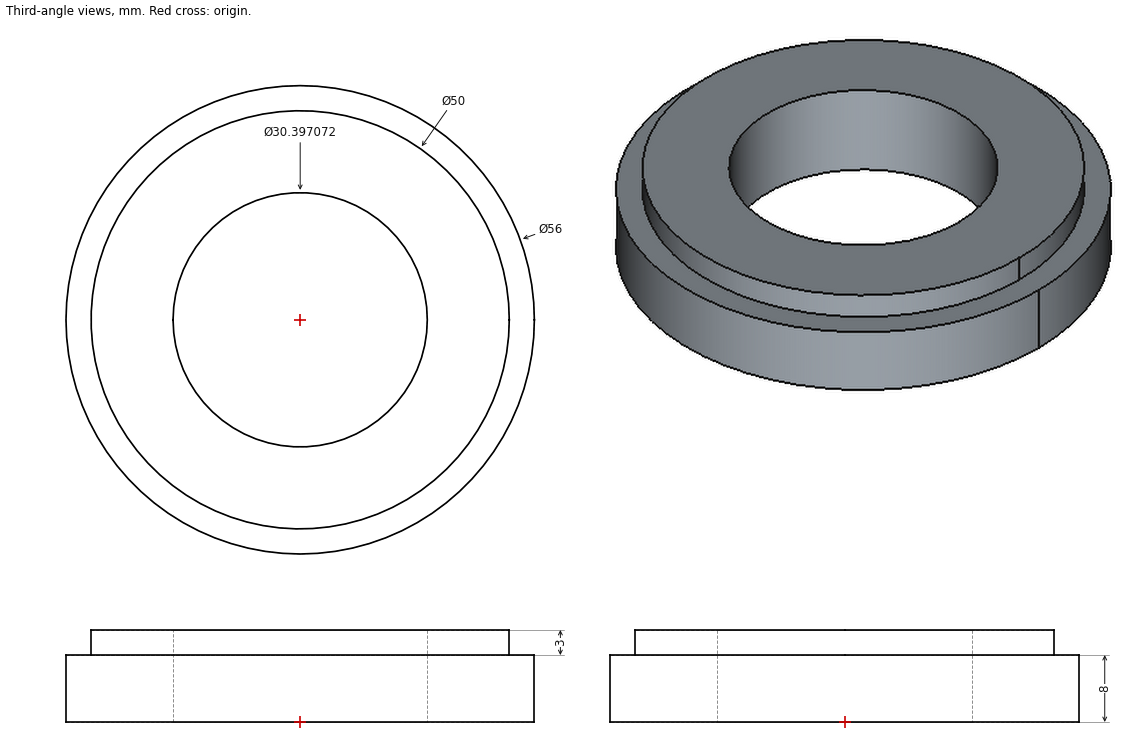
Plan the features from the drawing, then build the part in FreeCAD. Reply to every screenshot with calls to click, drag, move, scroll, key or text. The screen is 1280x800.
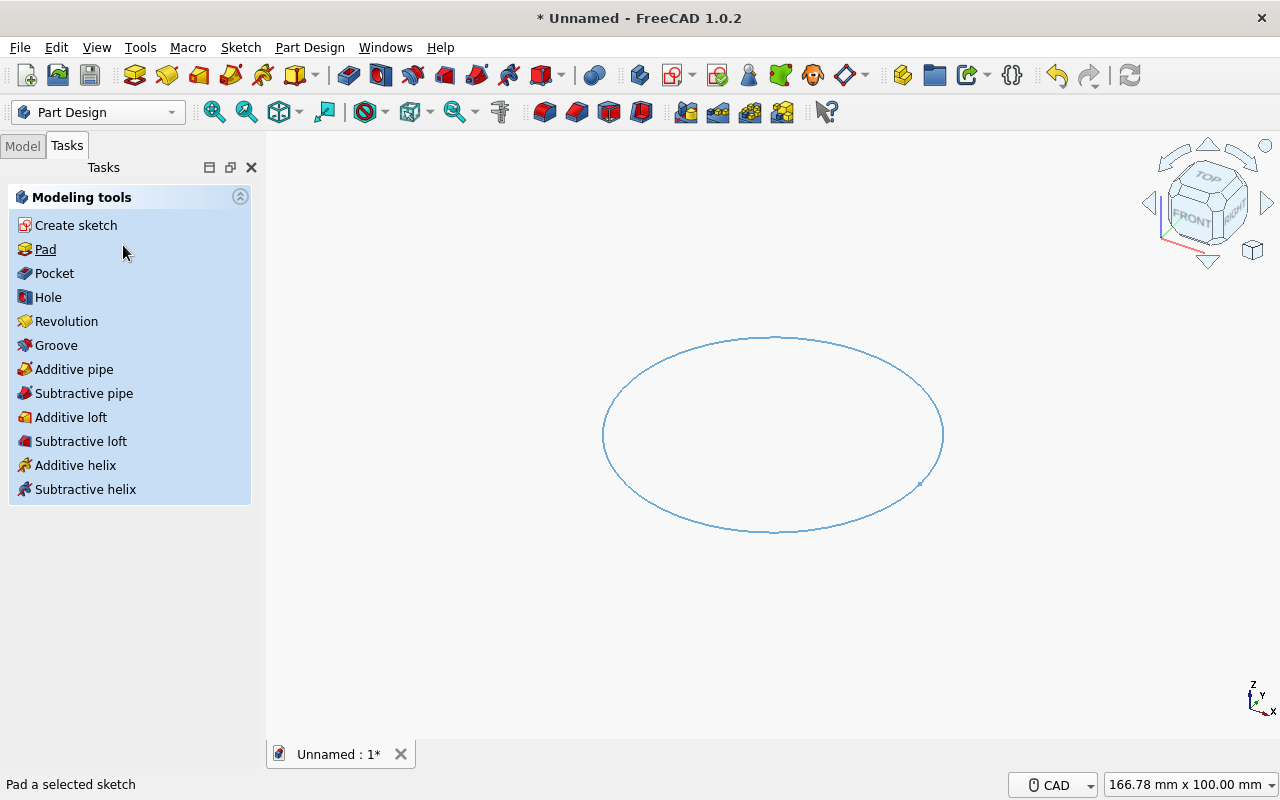
click(136, 76)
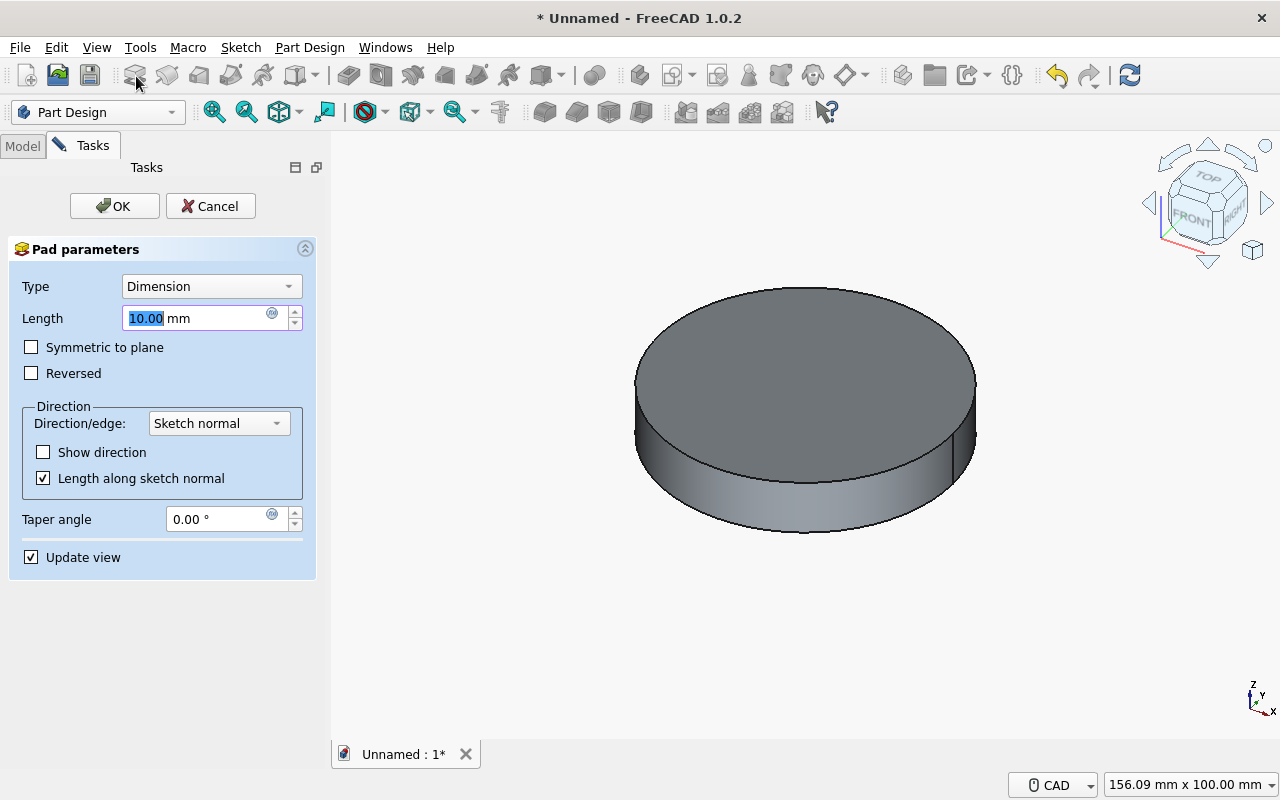
text(8)
key(Tab)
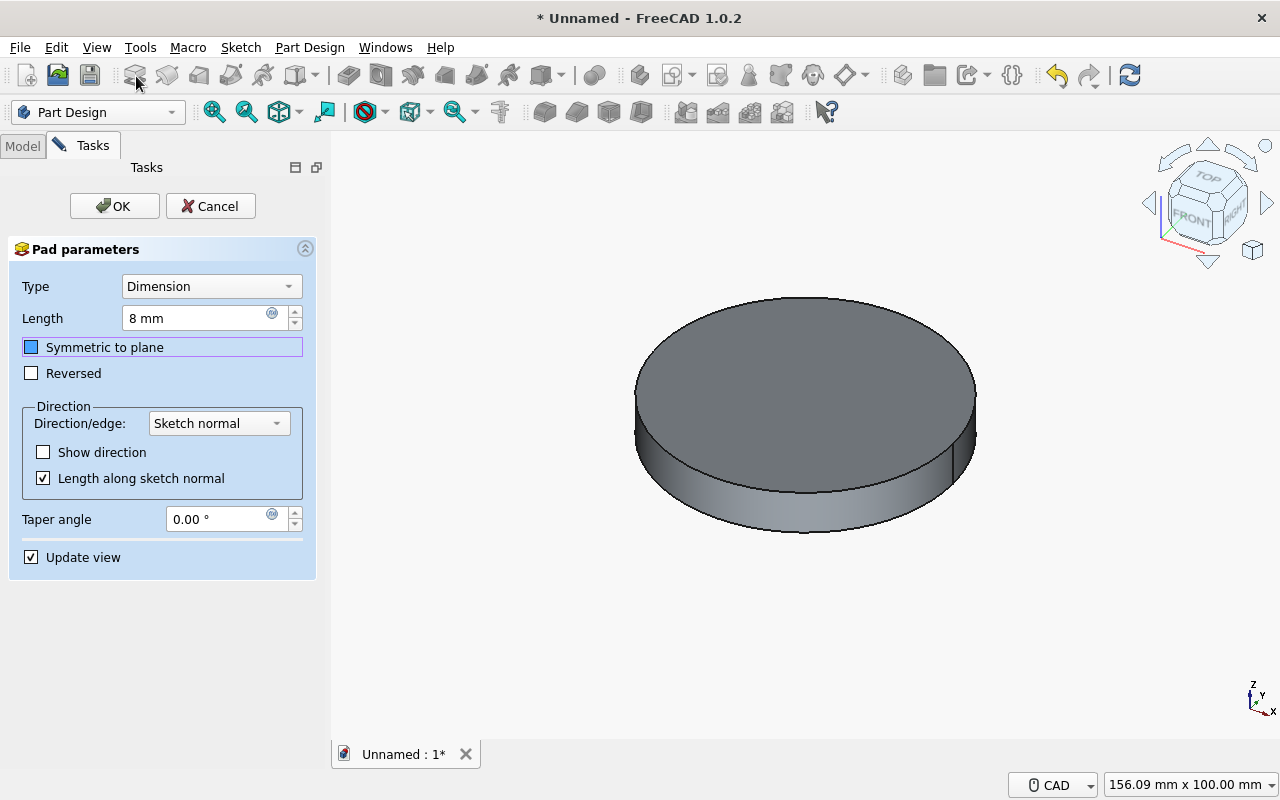
click(115, 206)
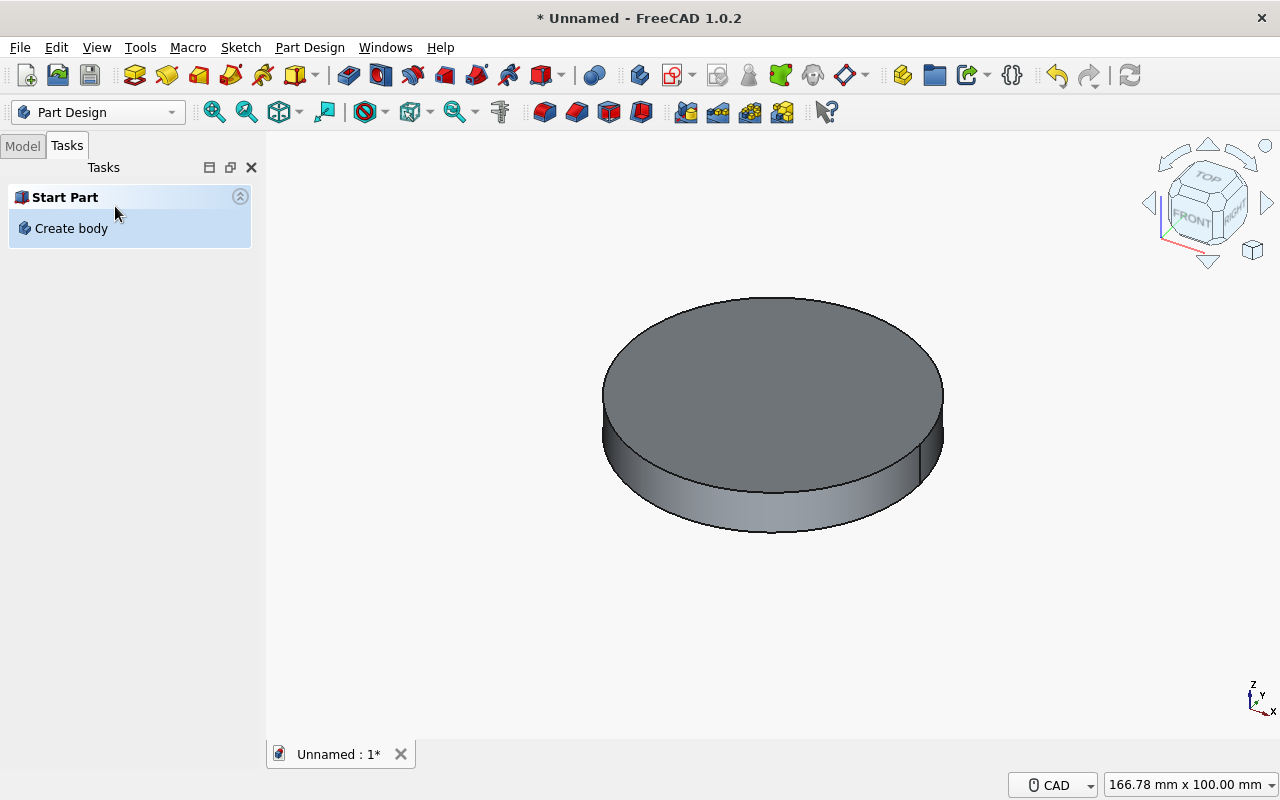
click(773, 394)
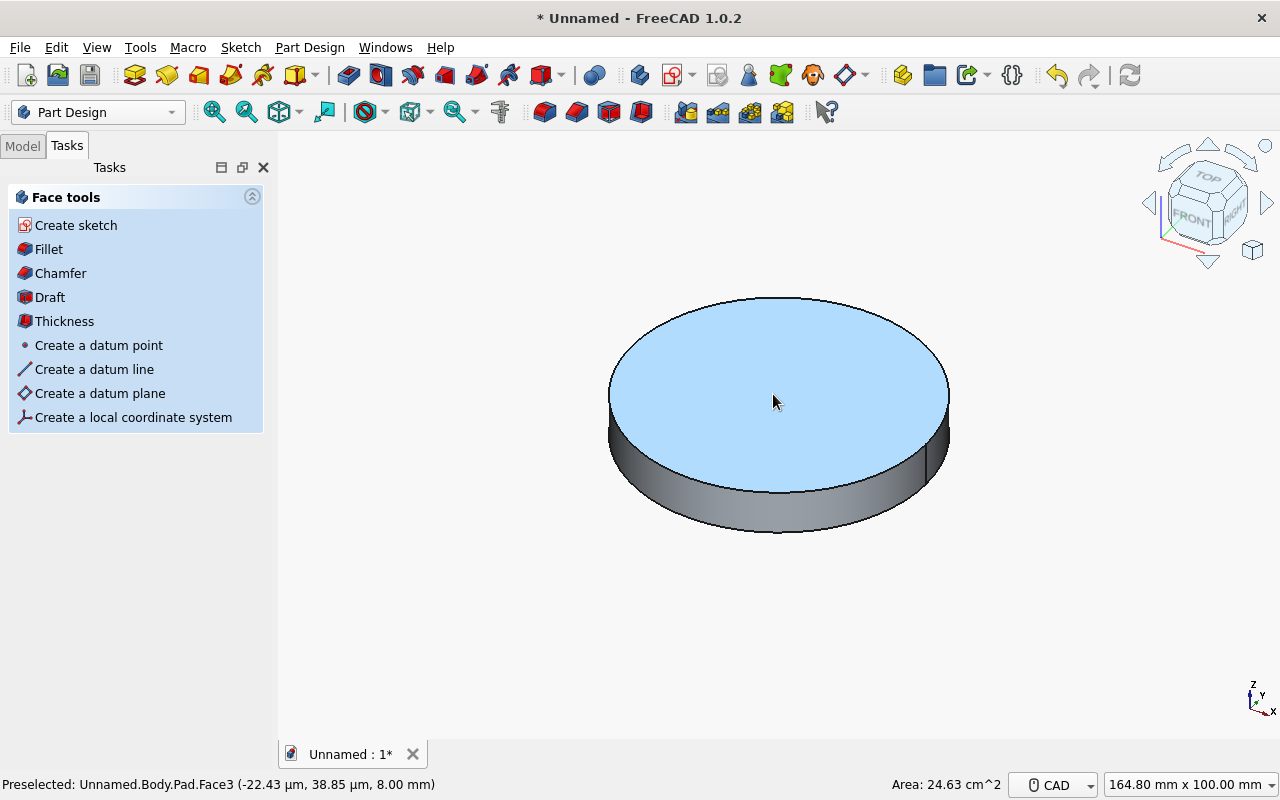
click(672, 76)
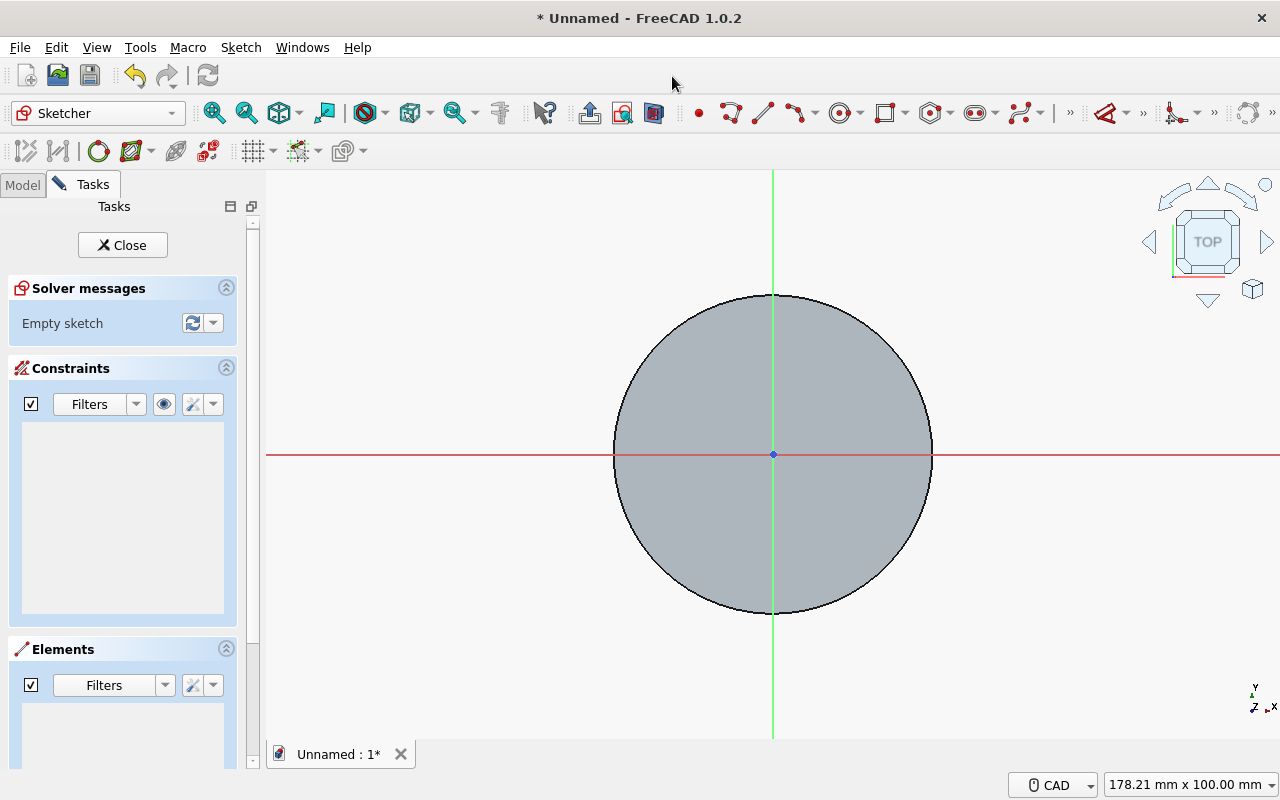
click(840, 114)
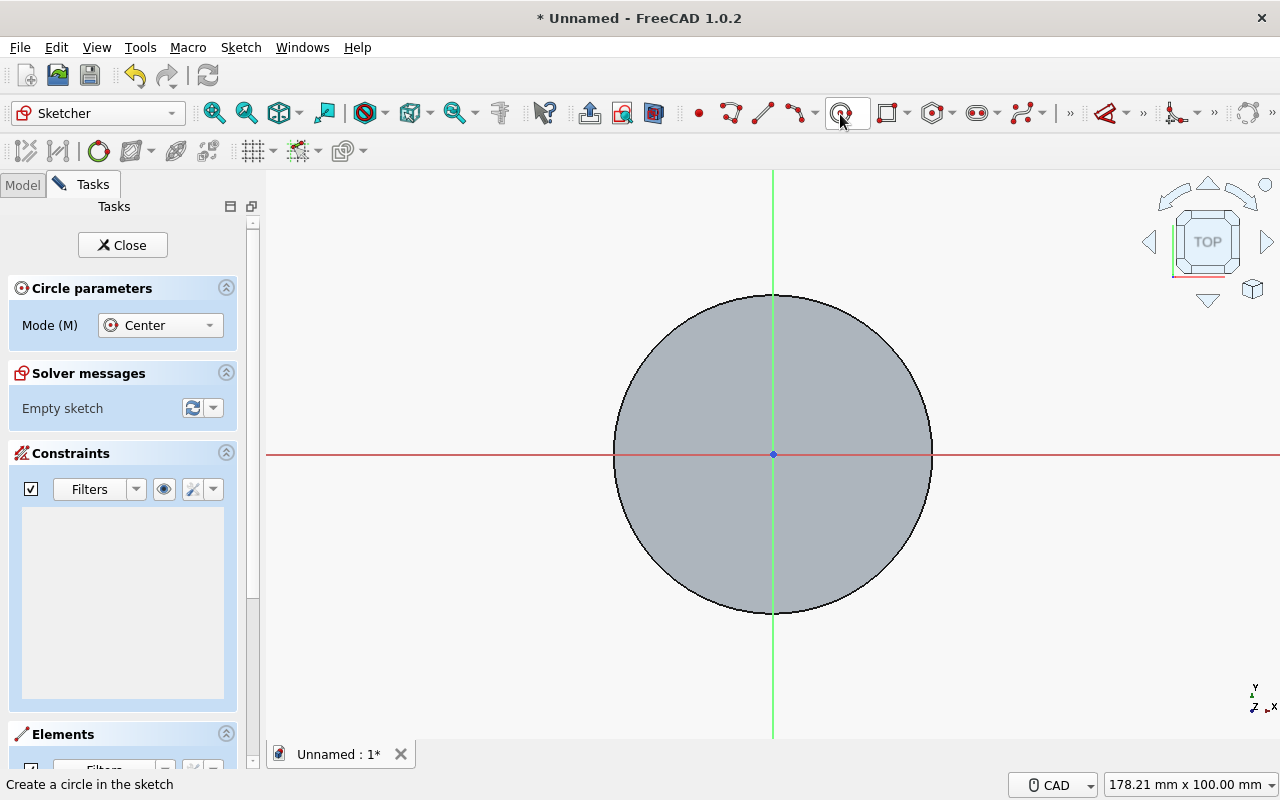
click(773, 454)
click(874, 354)
key(Escape)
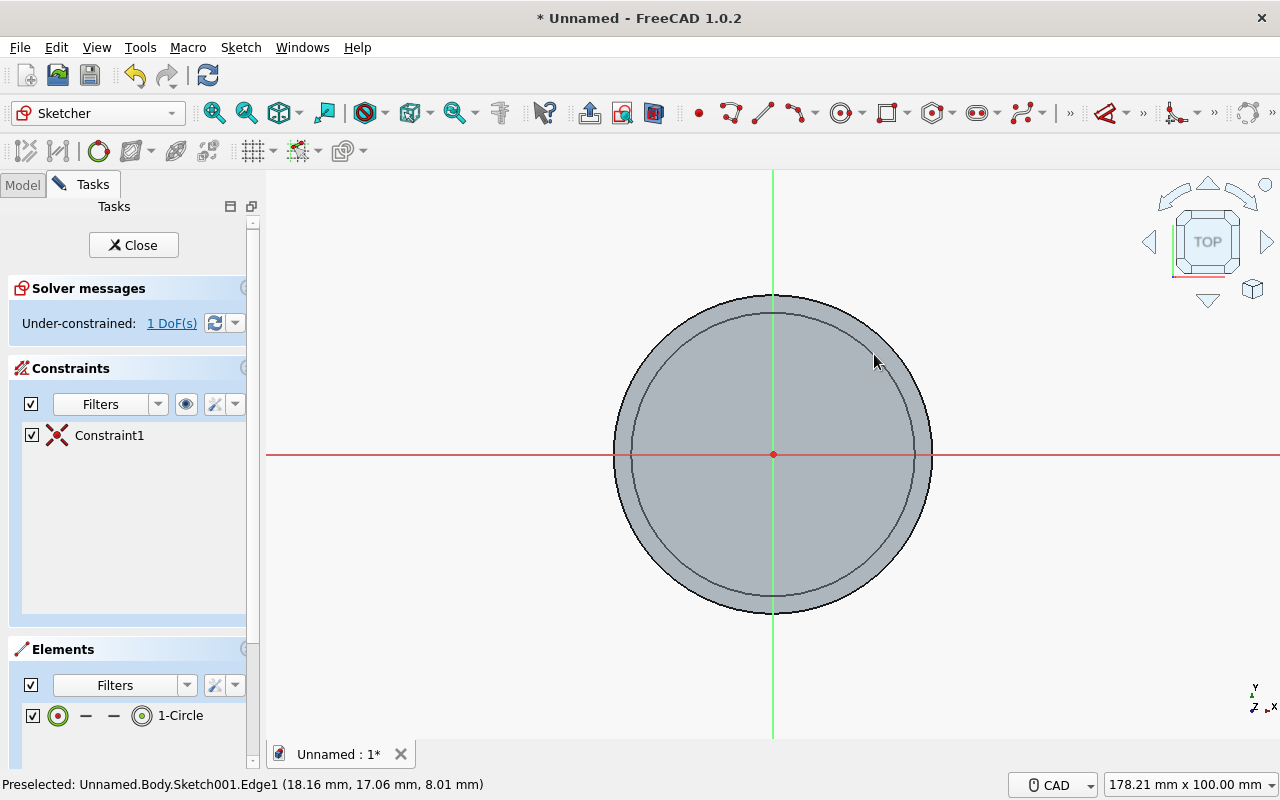
click(1106, 114)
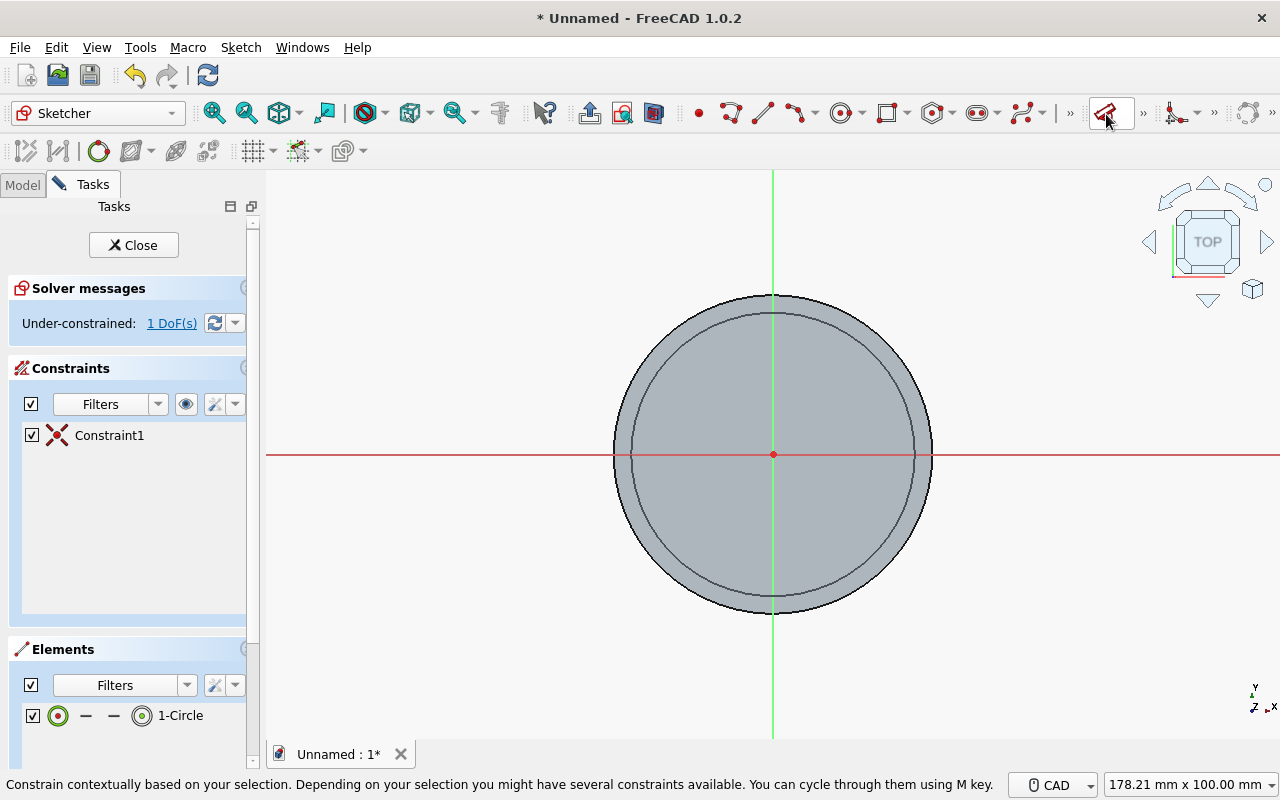
click(873, 354)
click(896, 331)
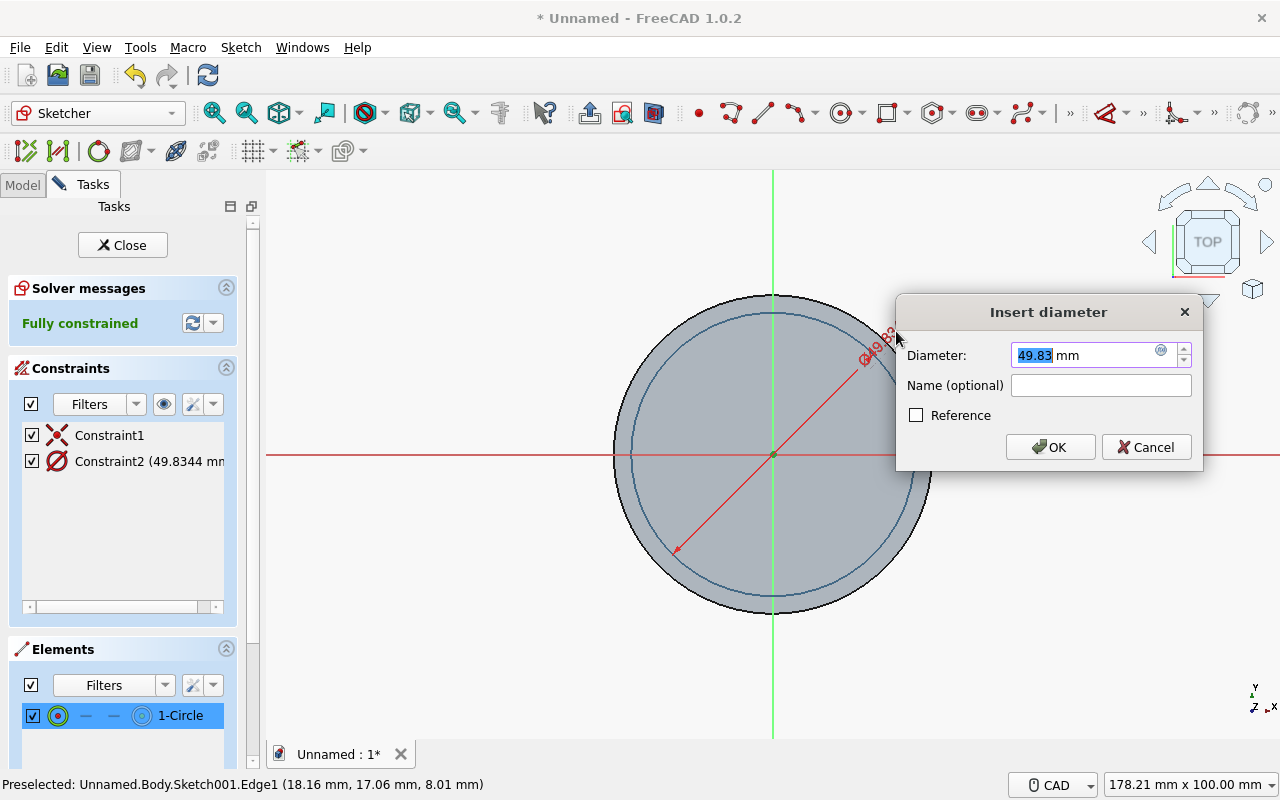
text(50)
key(Return)
key(Escape)